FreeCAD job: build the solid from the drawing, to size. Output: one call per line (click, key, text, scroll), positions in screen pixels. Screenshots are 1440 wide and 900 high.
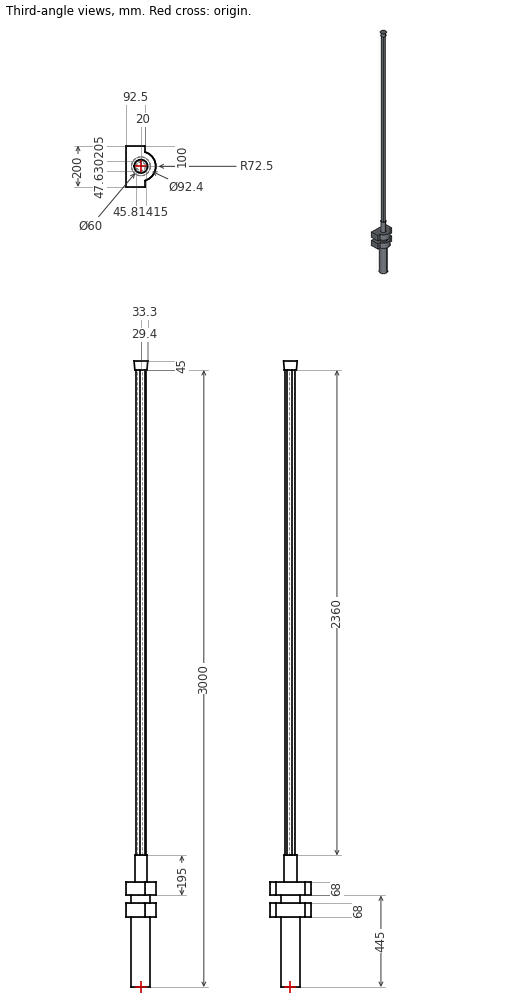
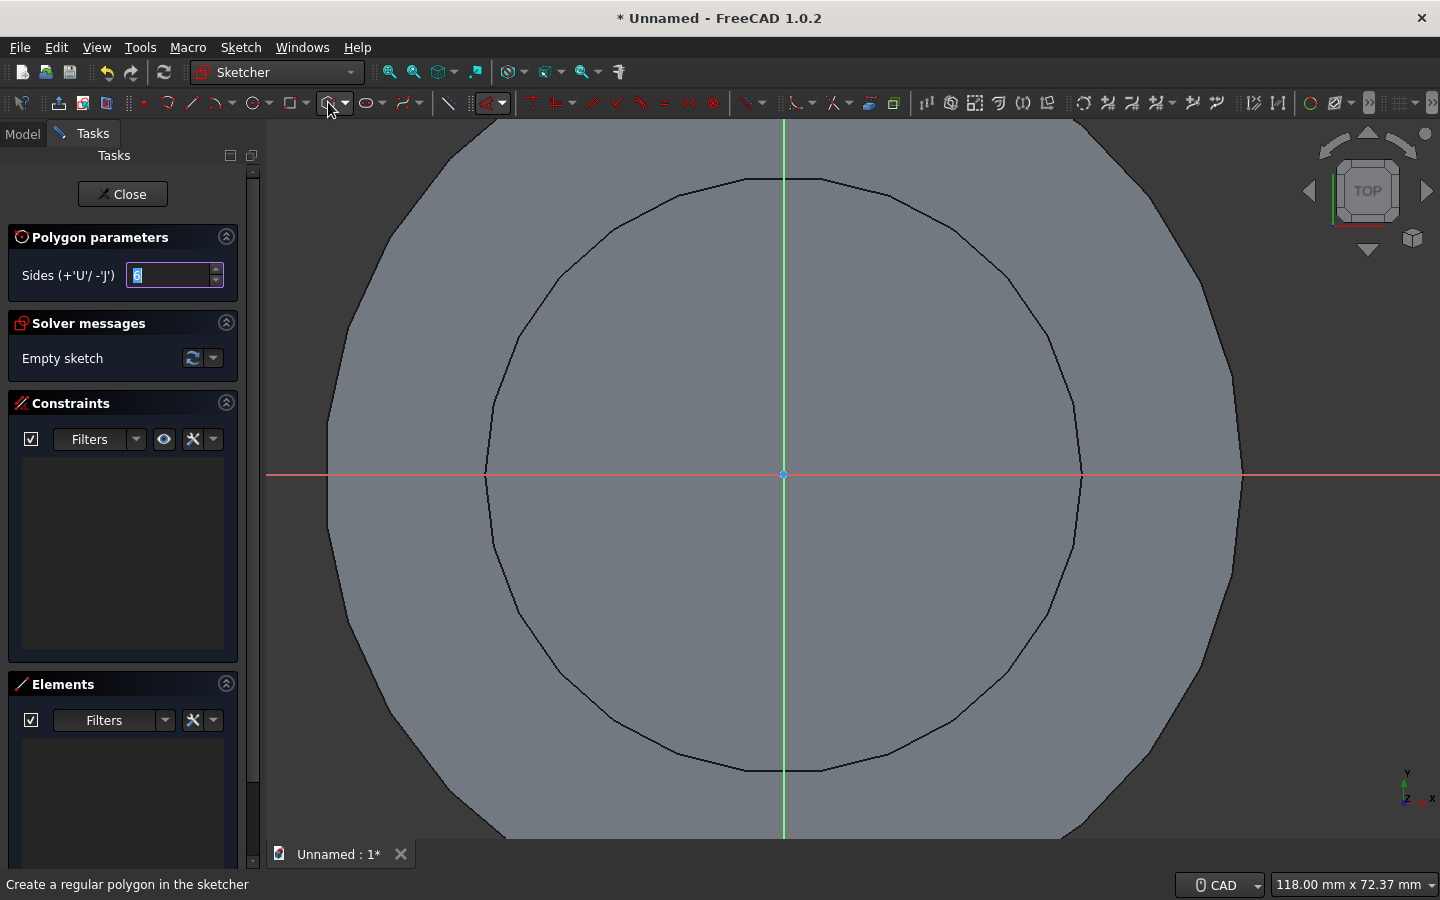
click(784, 475)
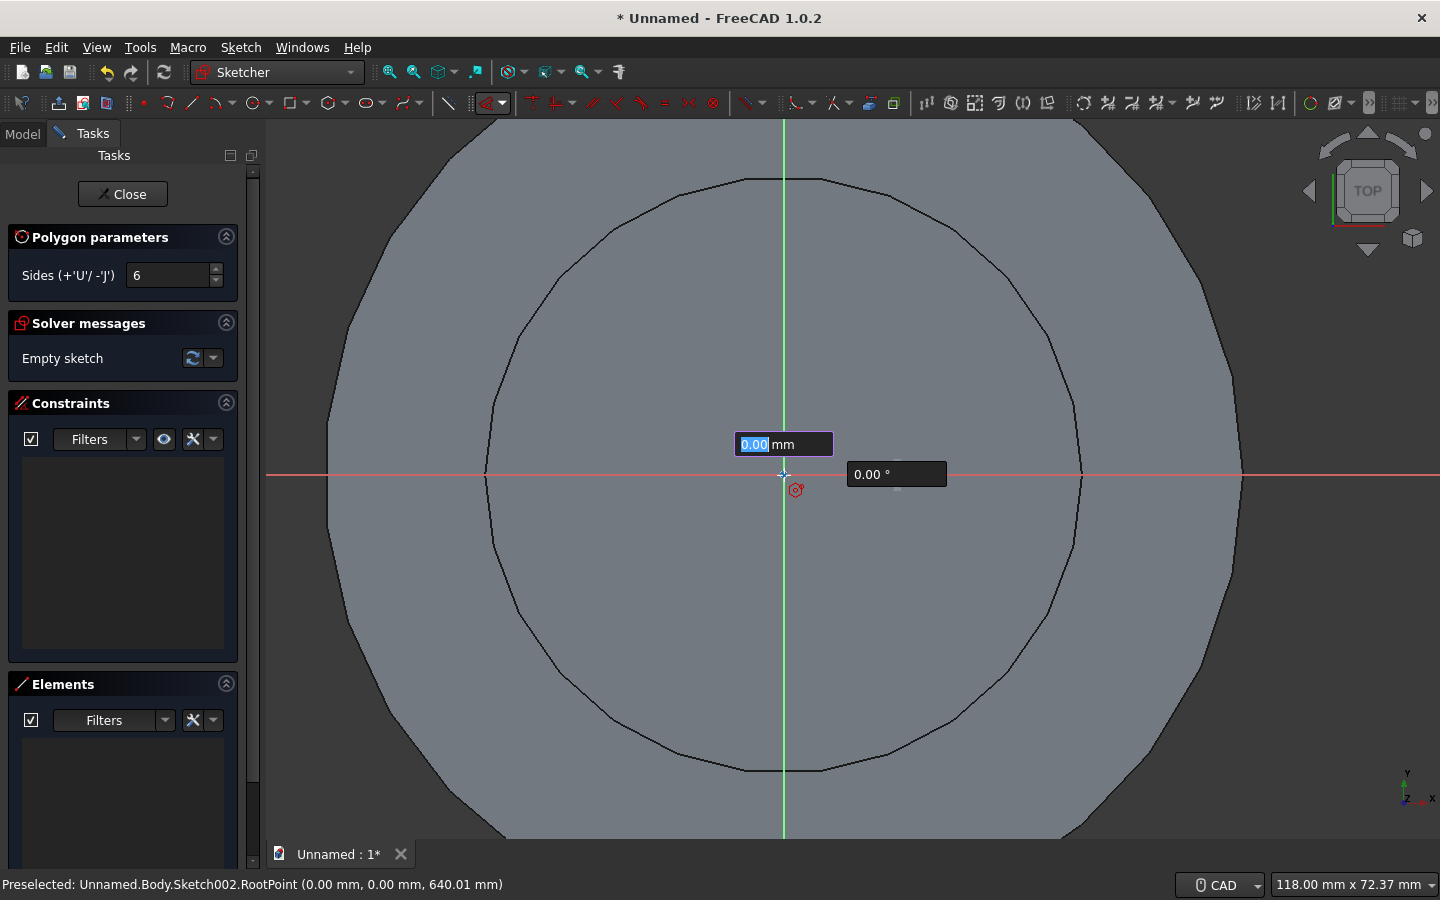
click(966, 633)
right_click(966, 633)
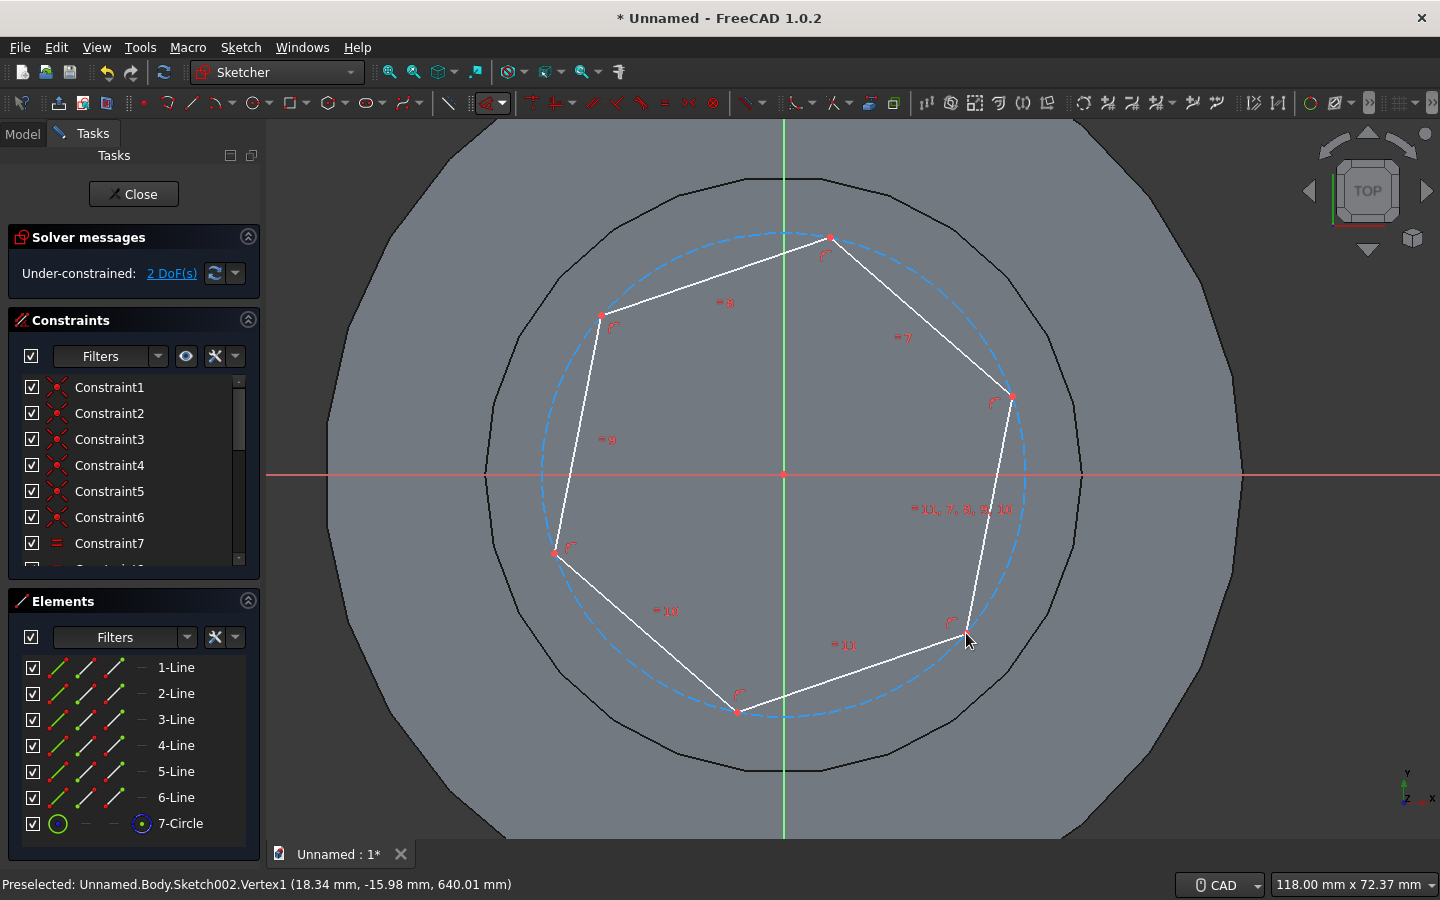
click(555, 553)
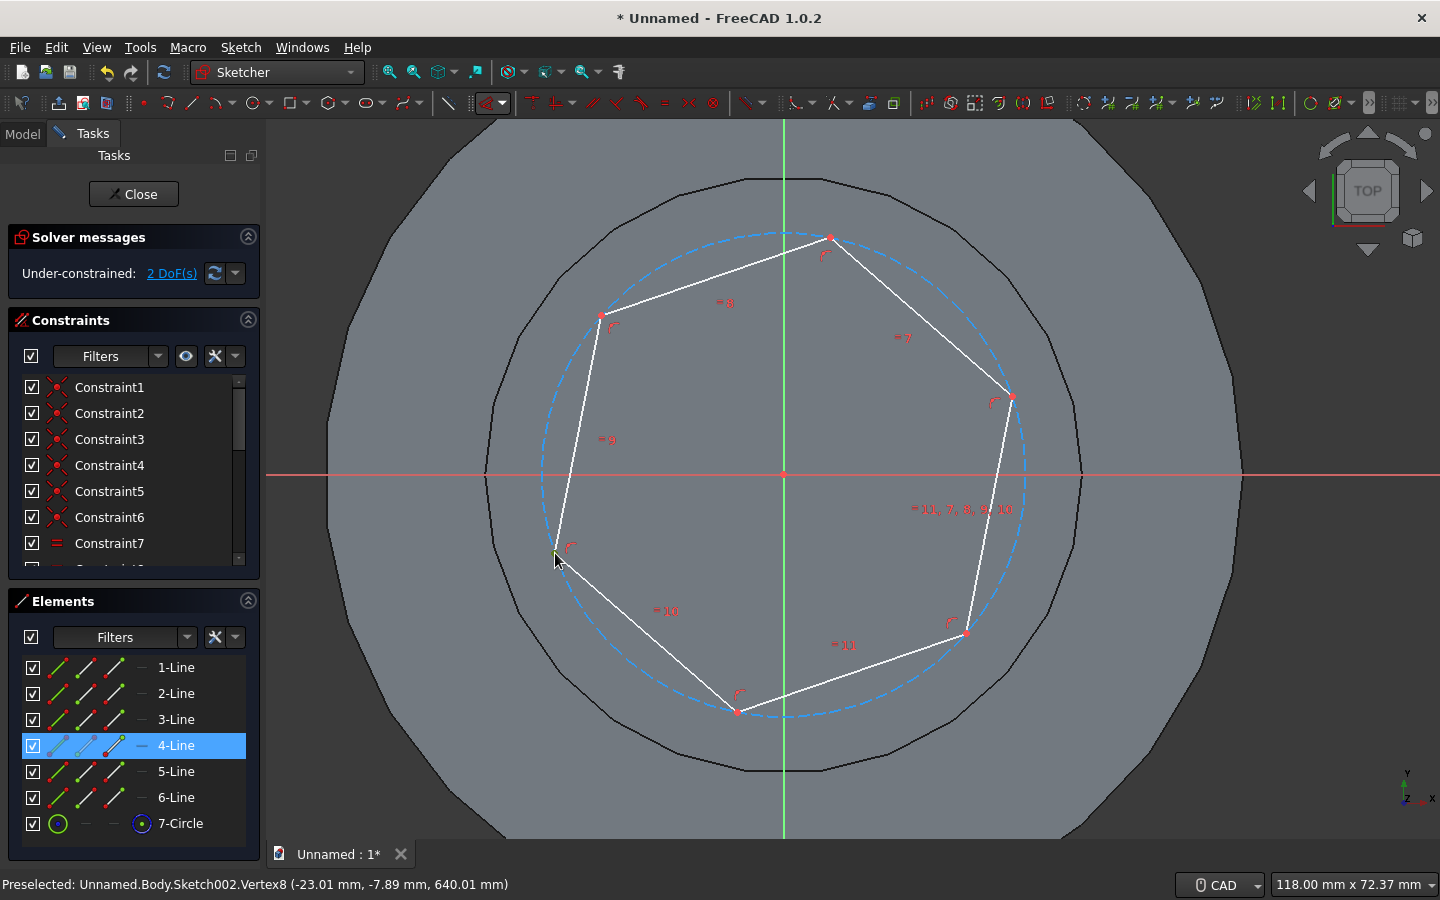
click(1012, 397)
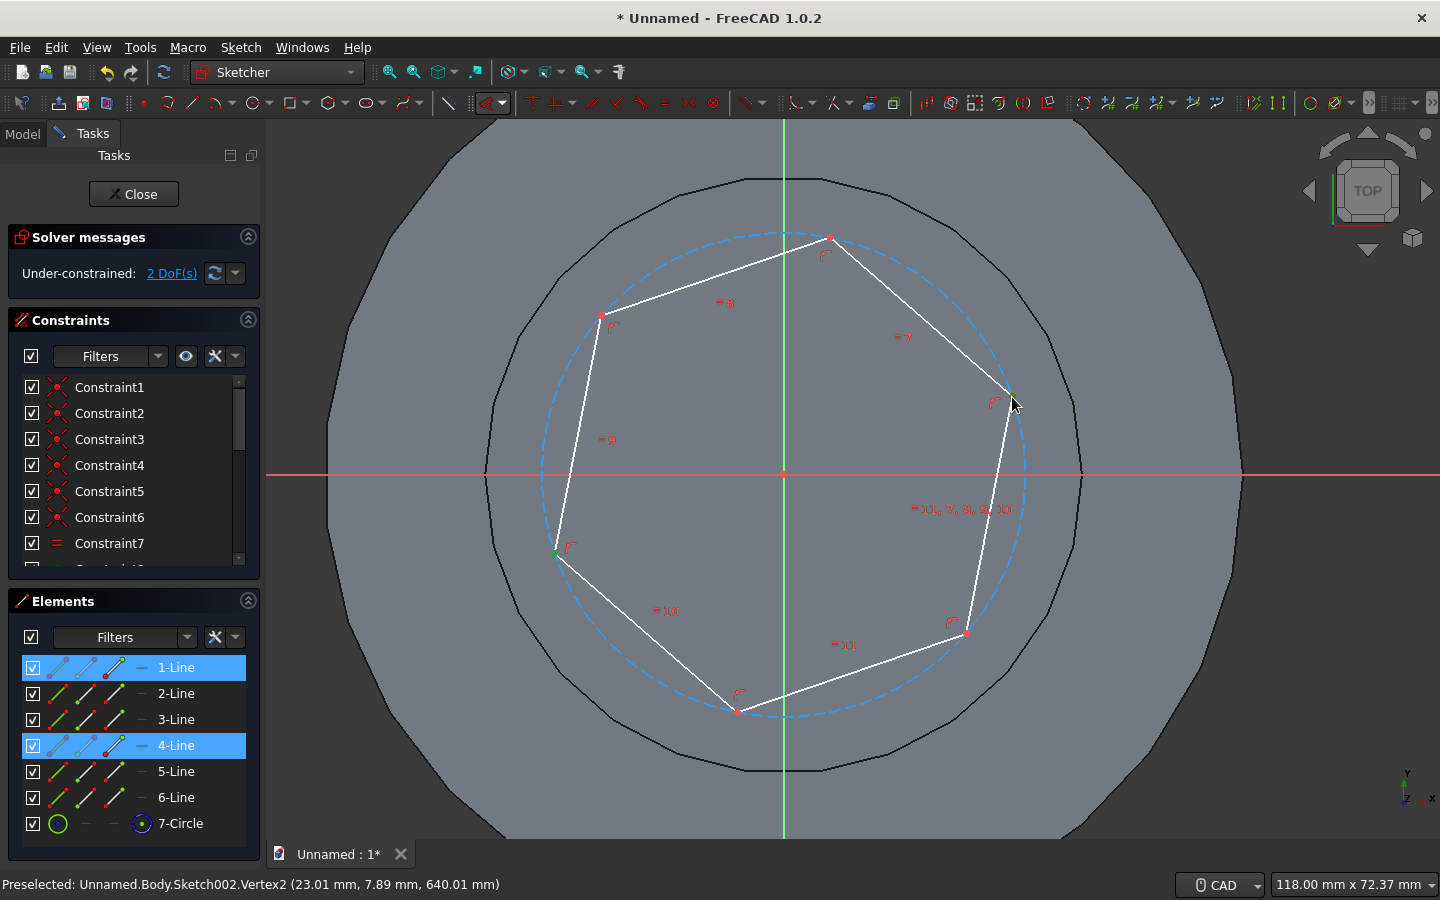
key(l)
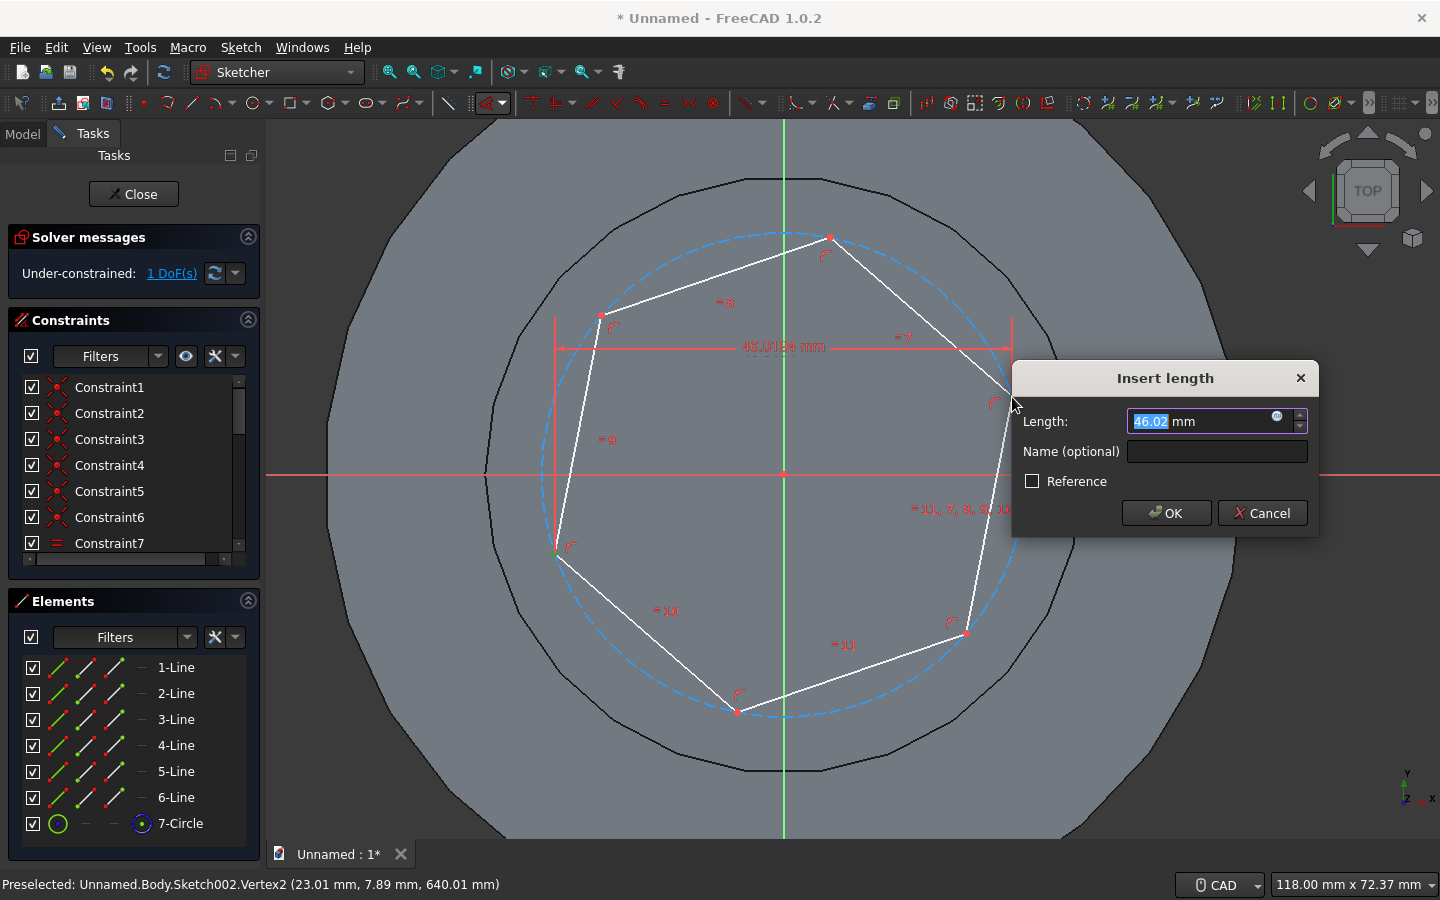
text(45.81415)
key(Return)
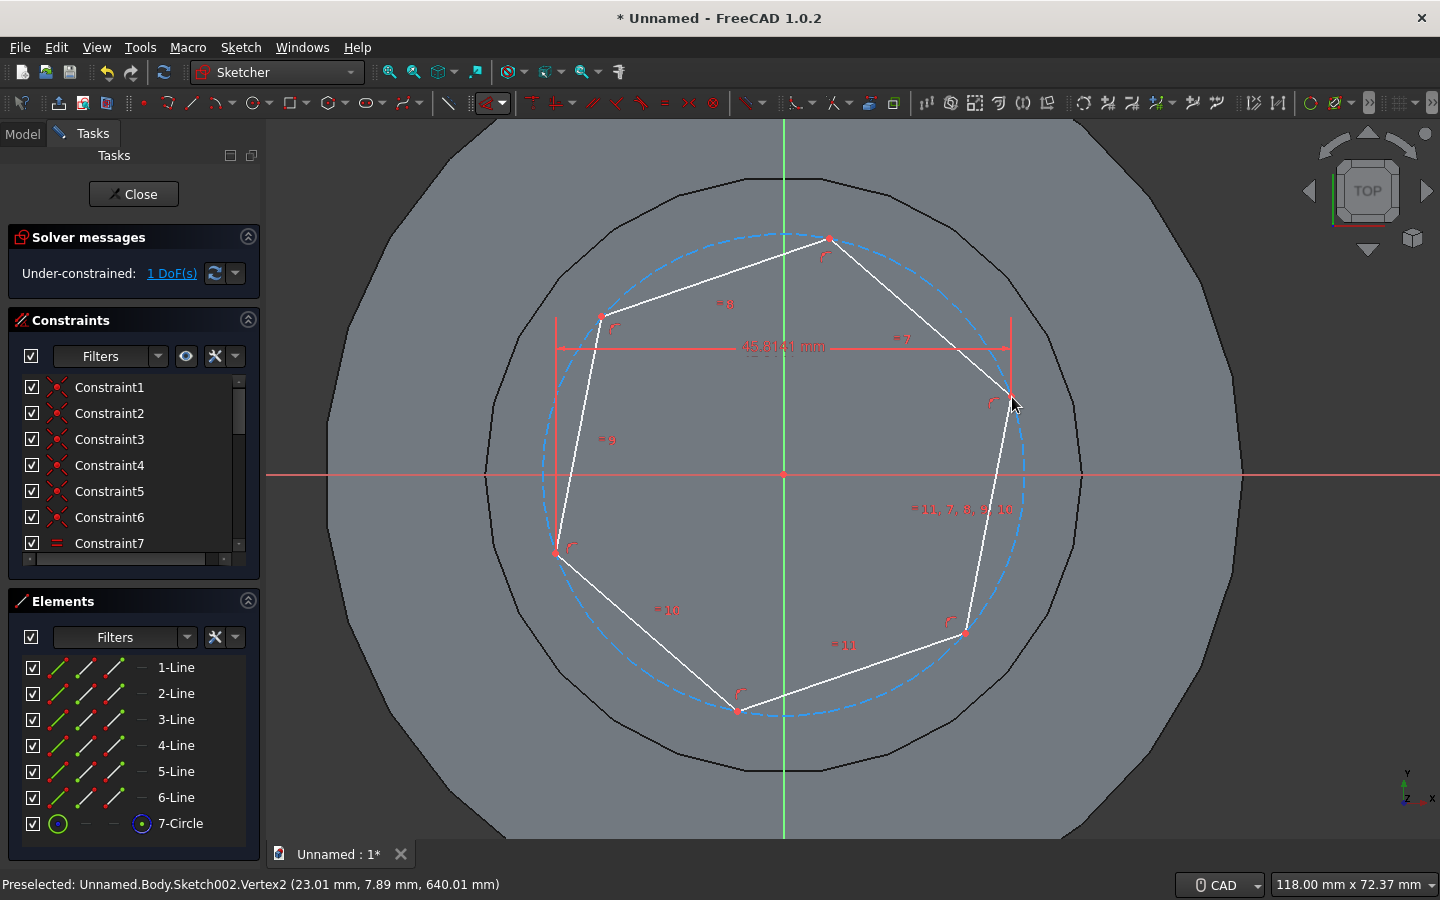
click(738, 712)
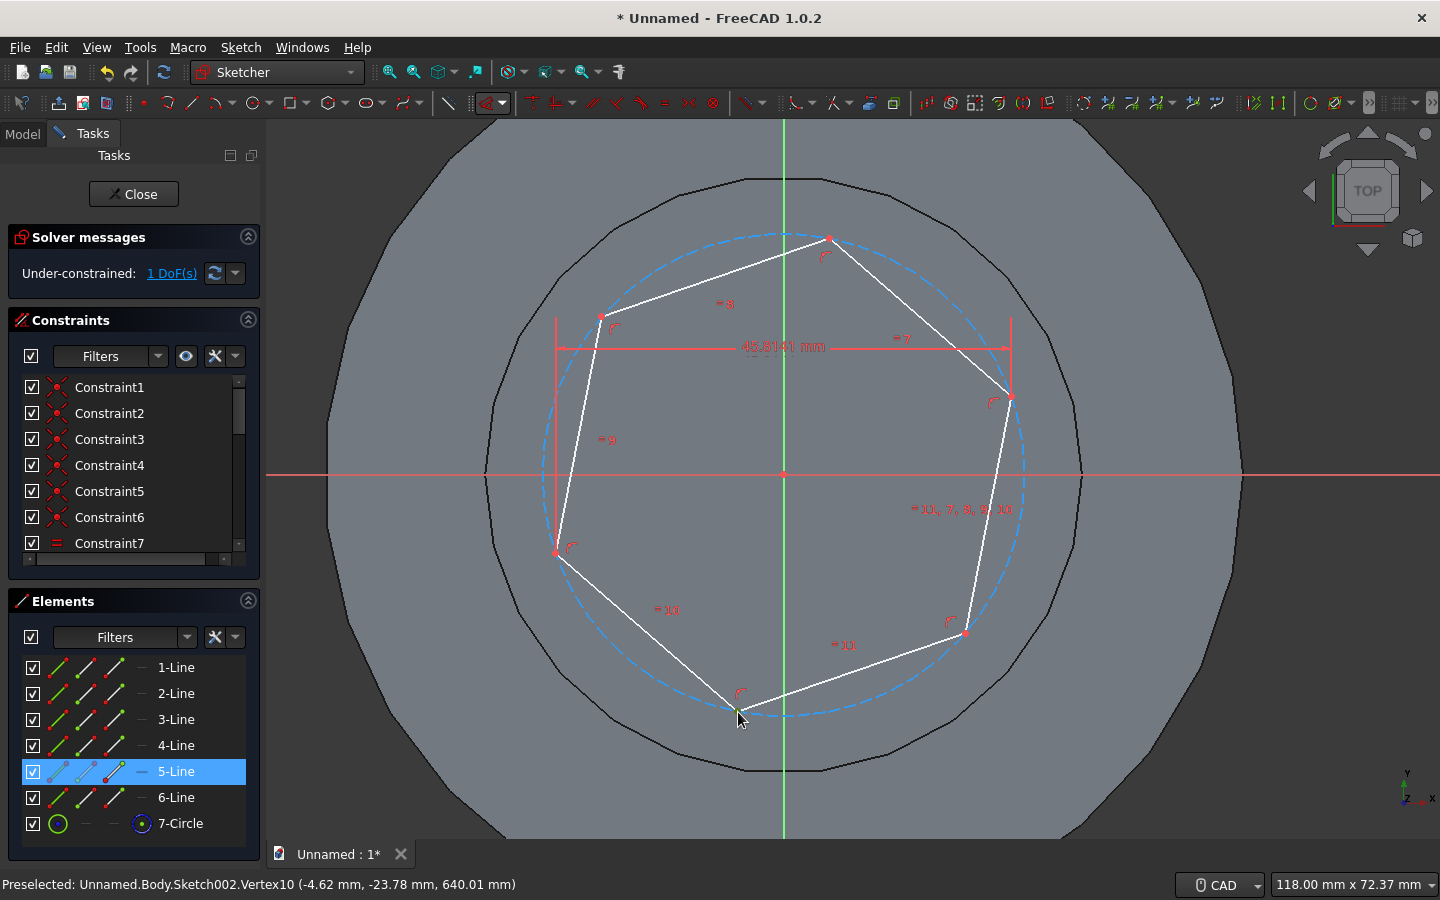
click(830, 238)